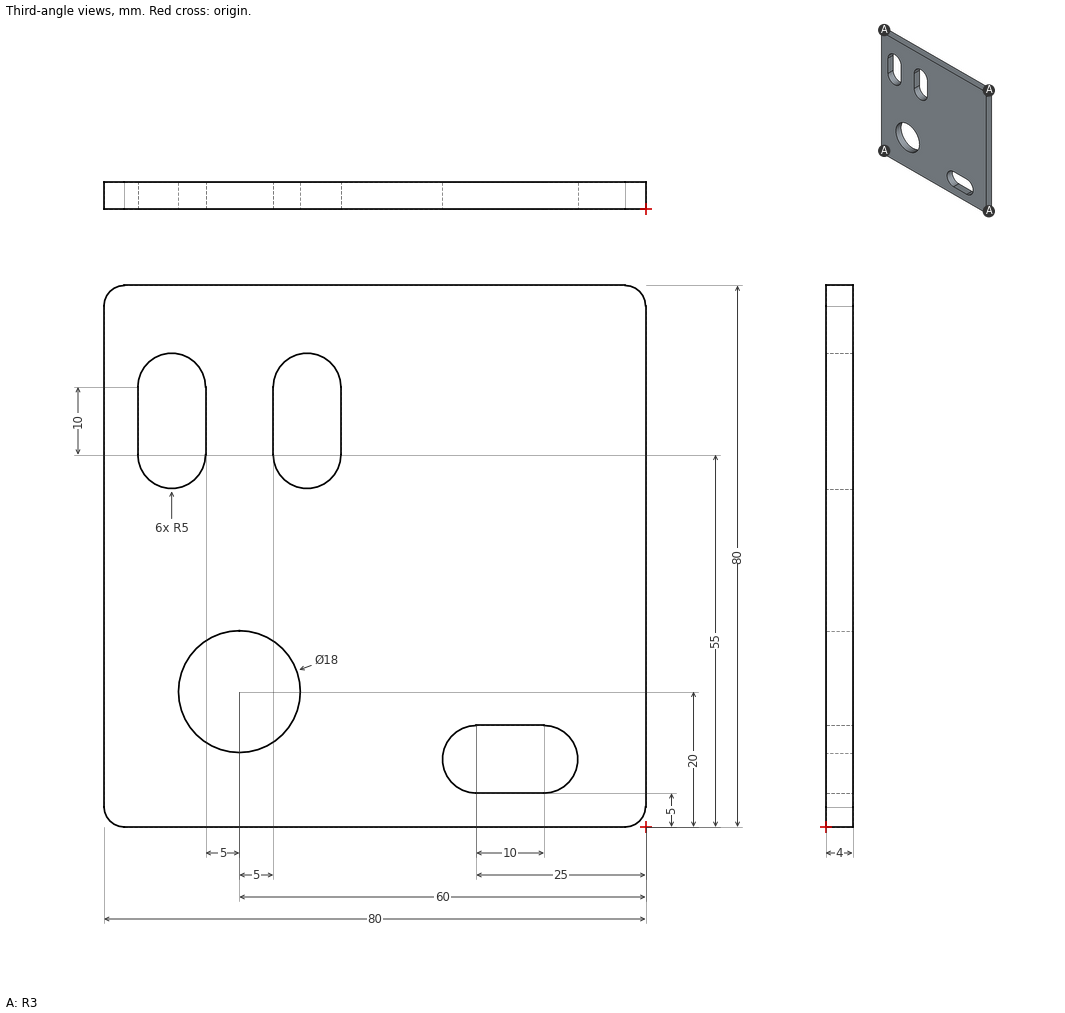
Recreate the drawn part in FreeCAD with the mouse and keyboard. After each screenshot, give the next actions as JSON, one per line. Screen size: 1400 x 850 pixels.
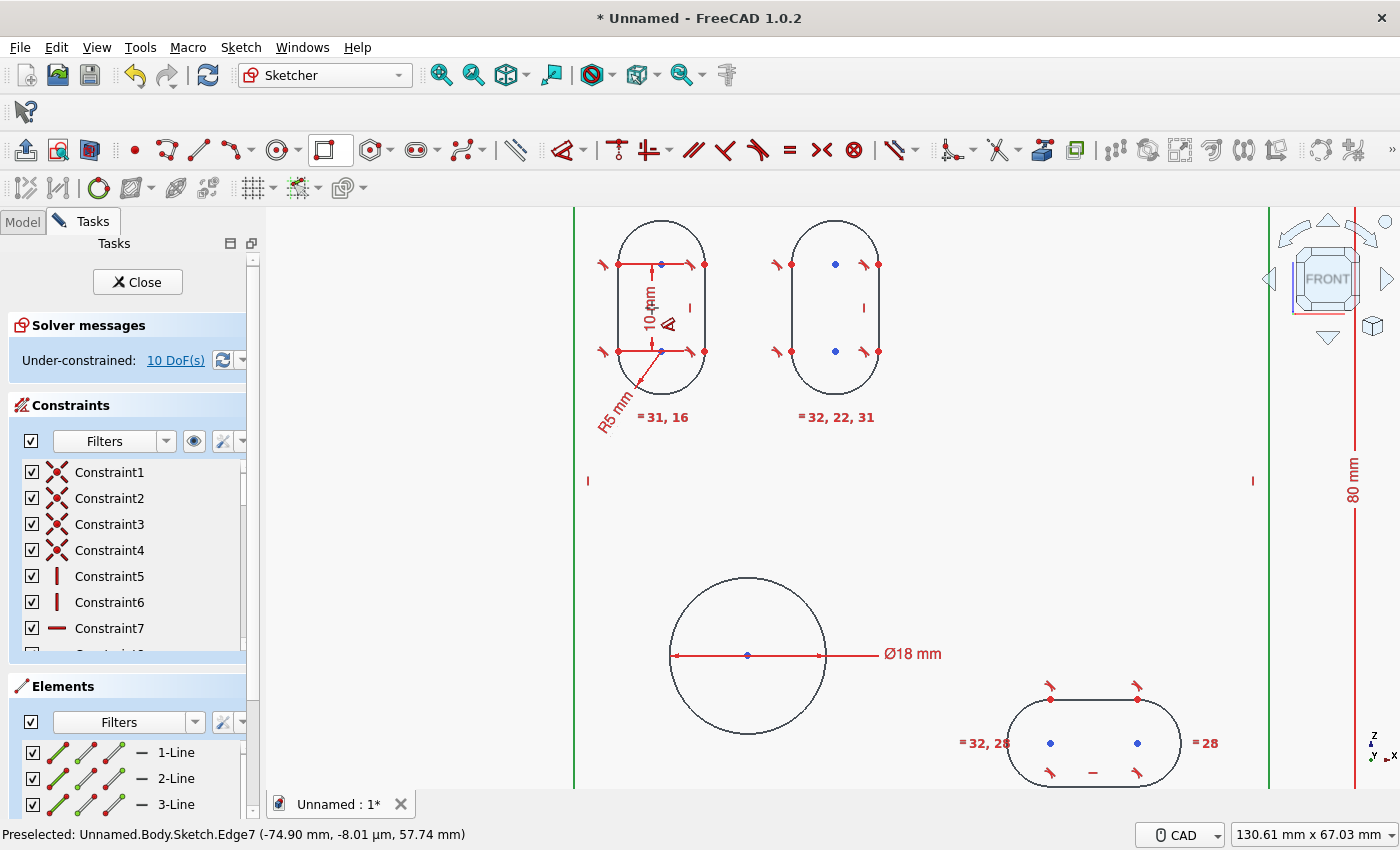
{"action": "left_click", "coordinate": [792, 325]}
{"action": "left_click", "coordinate": [758, 308]}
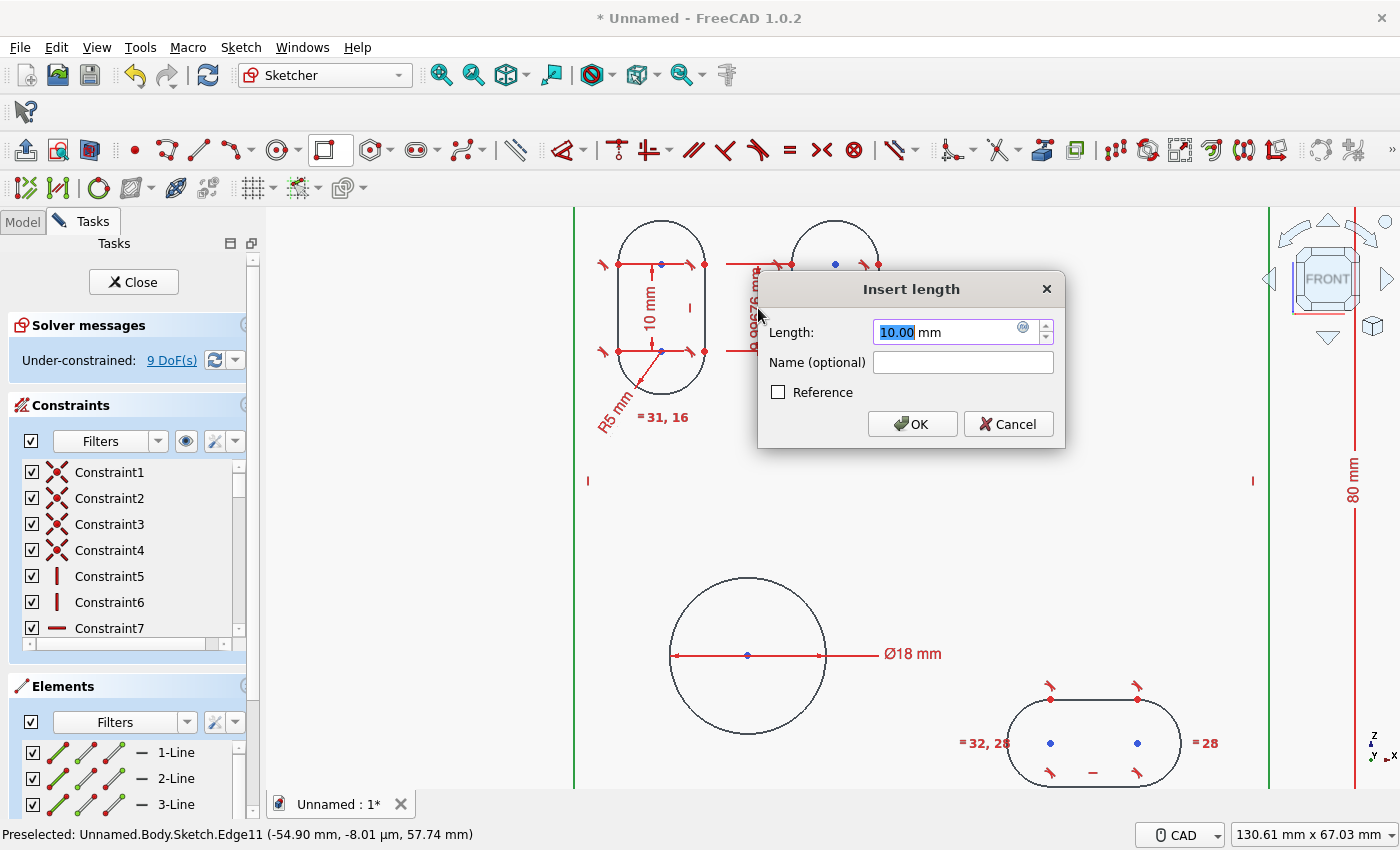
{"action": "type", "text": "10"}
{"action": "key", "text": "Return"}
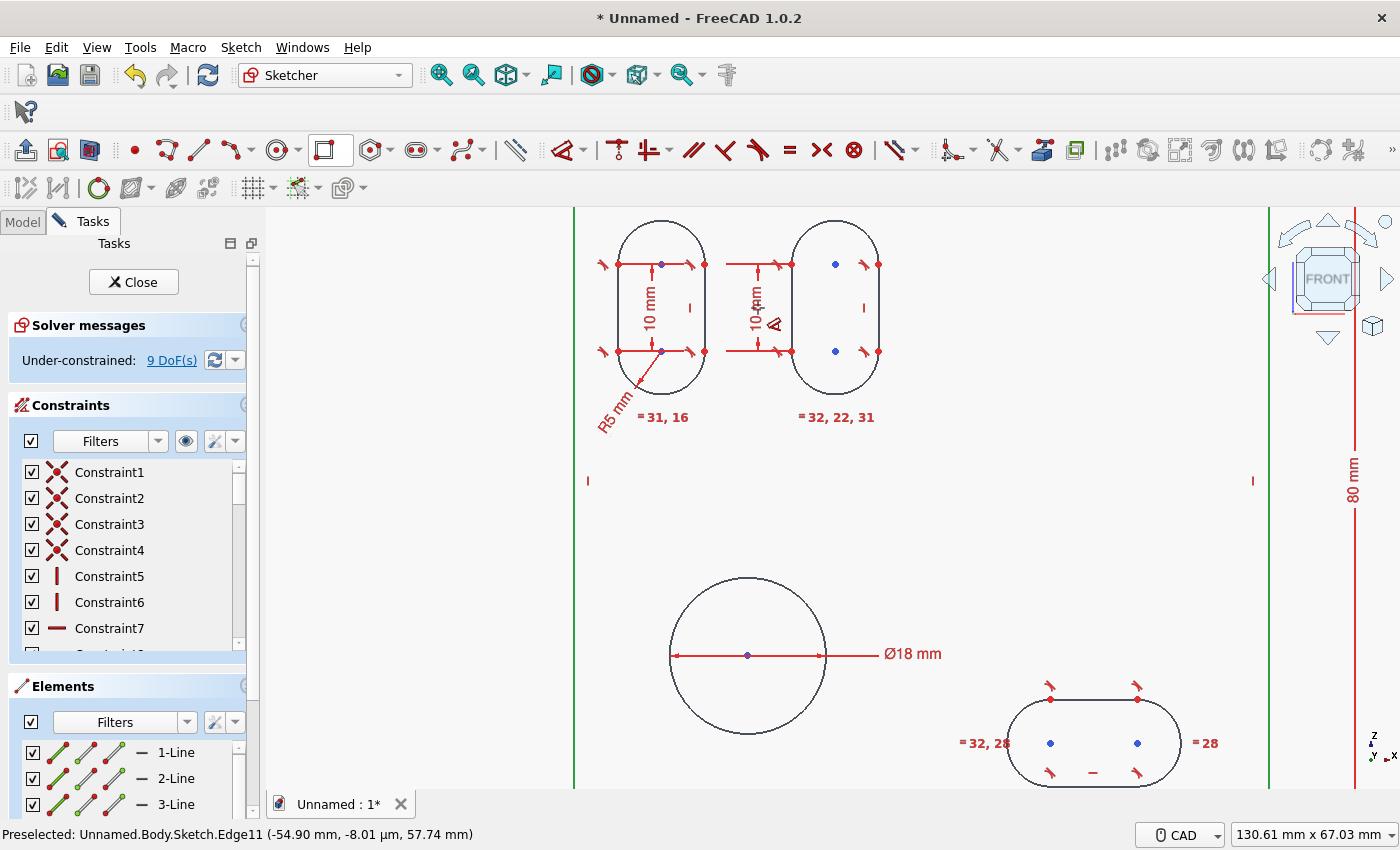
{"action": "left_click", "coordinate": [1077, 700]}
{"action": "left_click", "coordinate": [1094, 734]}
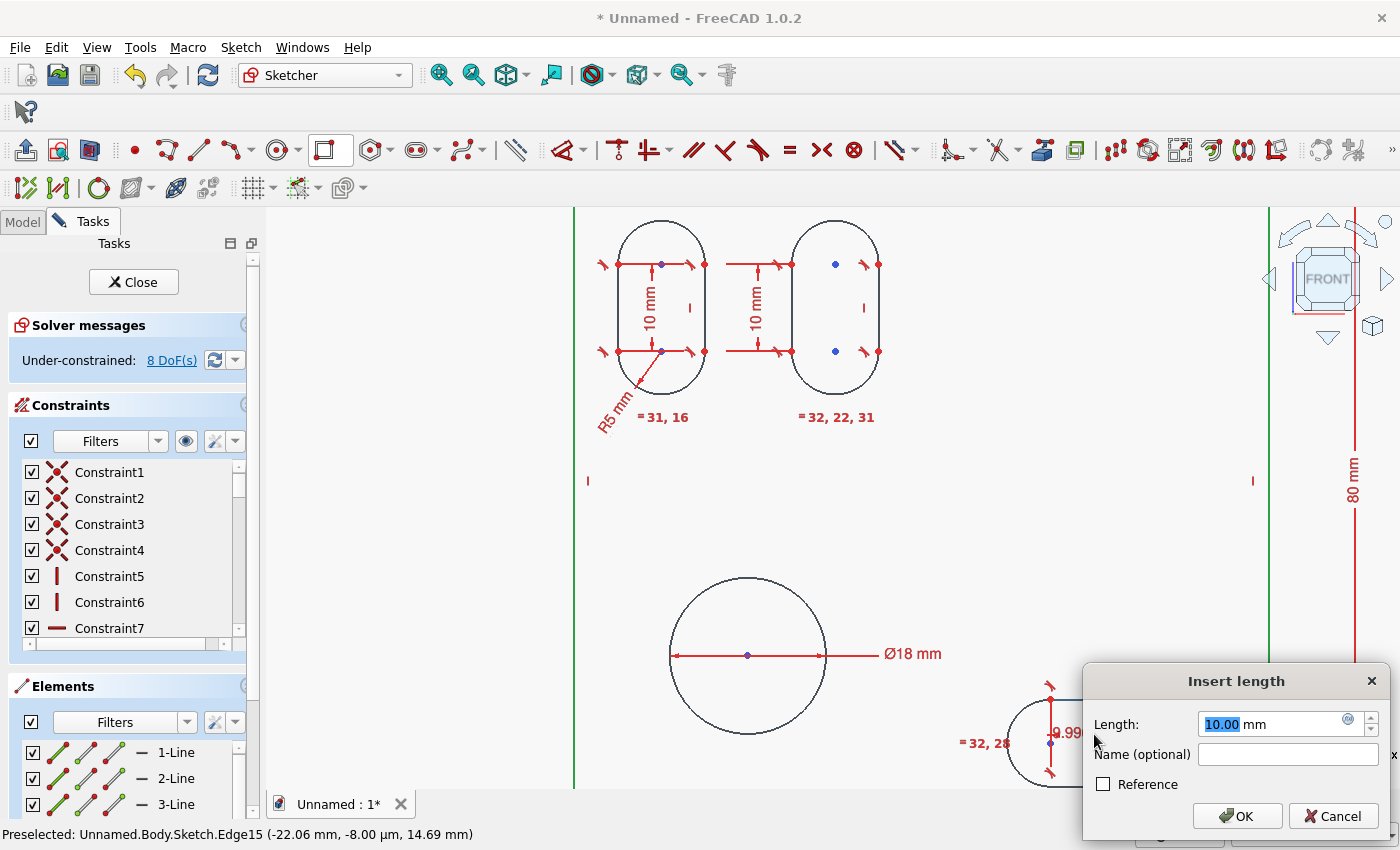
{"action": "type", "text": "10"}
{"action": "key", "text": "Return"}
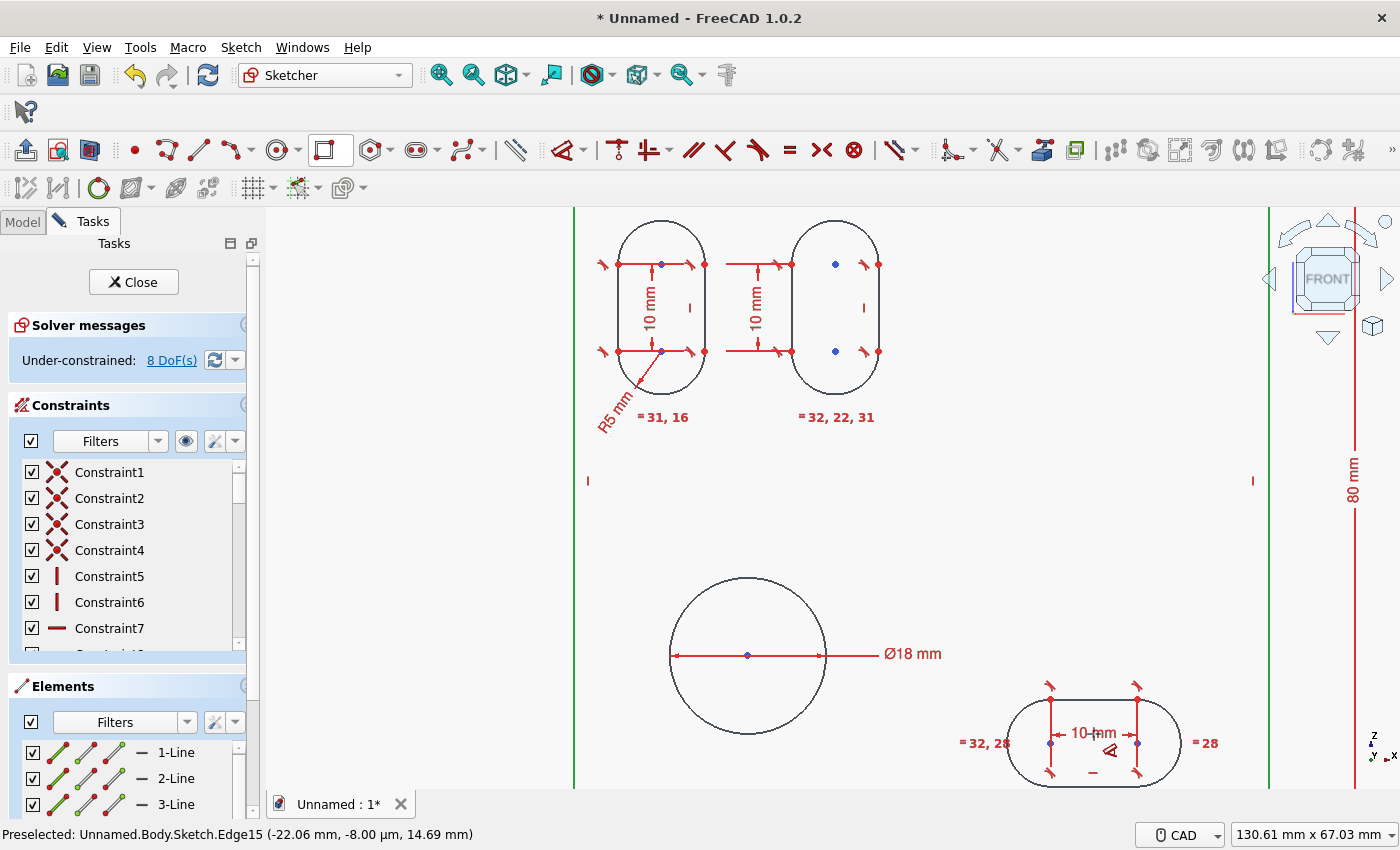
{"action": "scroll", "coordinate": [574, 520], "scroll_direction": "down", "scroll_amount": 3}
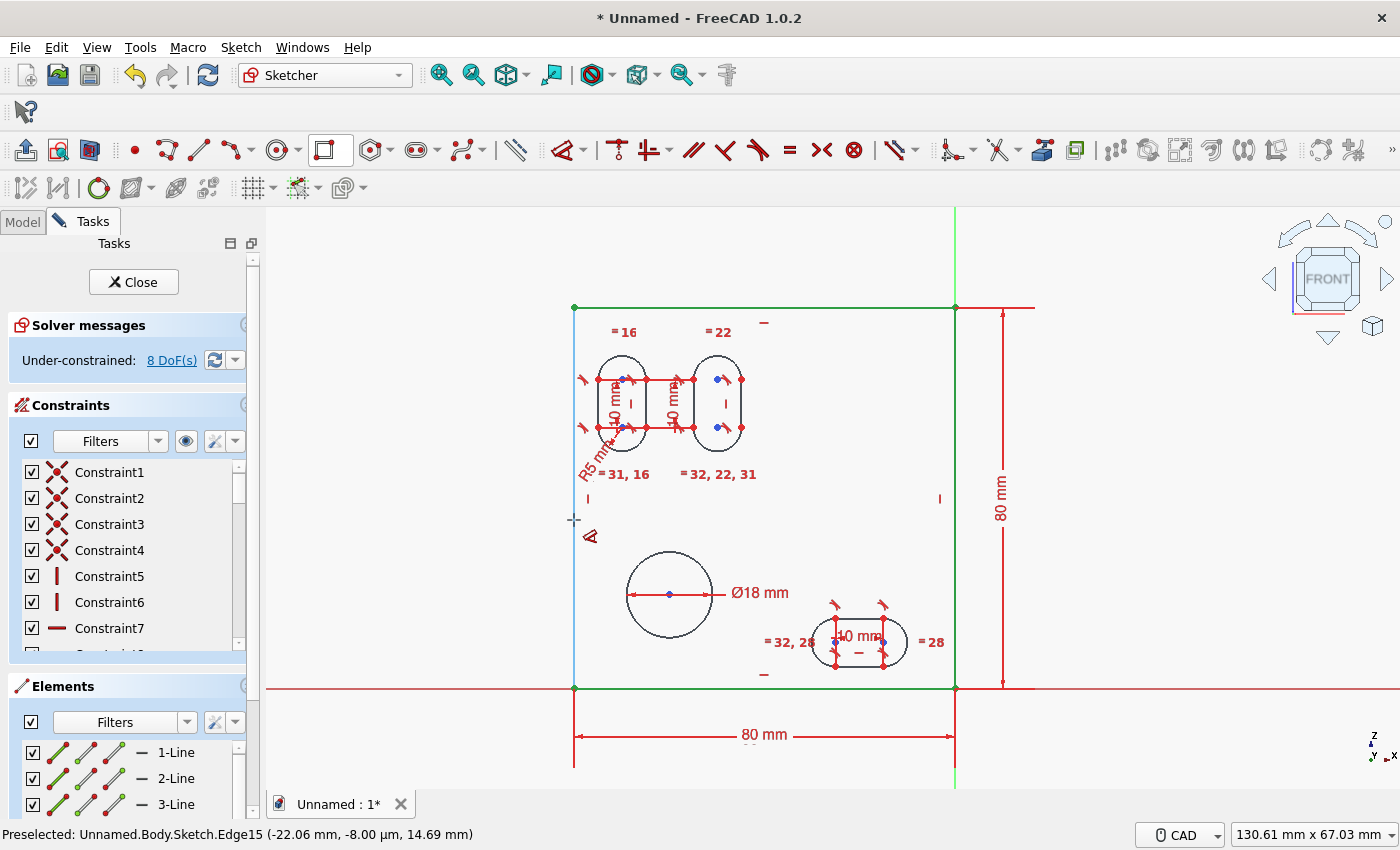
{"action": "scroll", "coordinate": [836, 667], "scroll_direction": "up", "scroll_amount": 3}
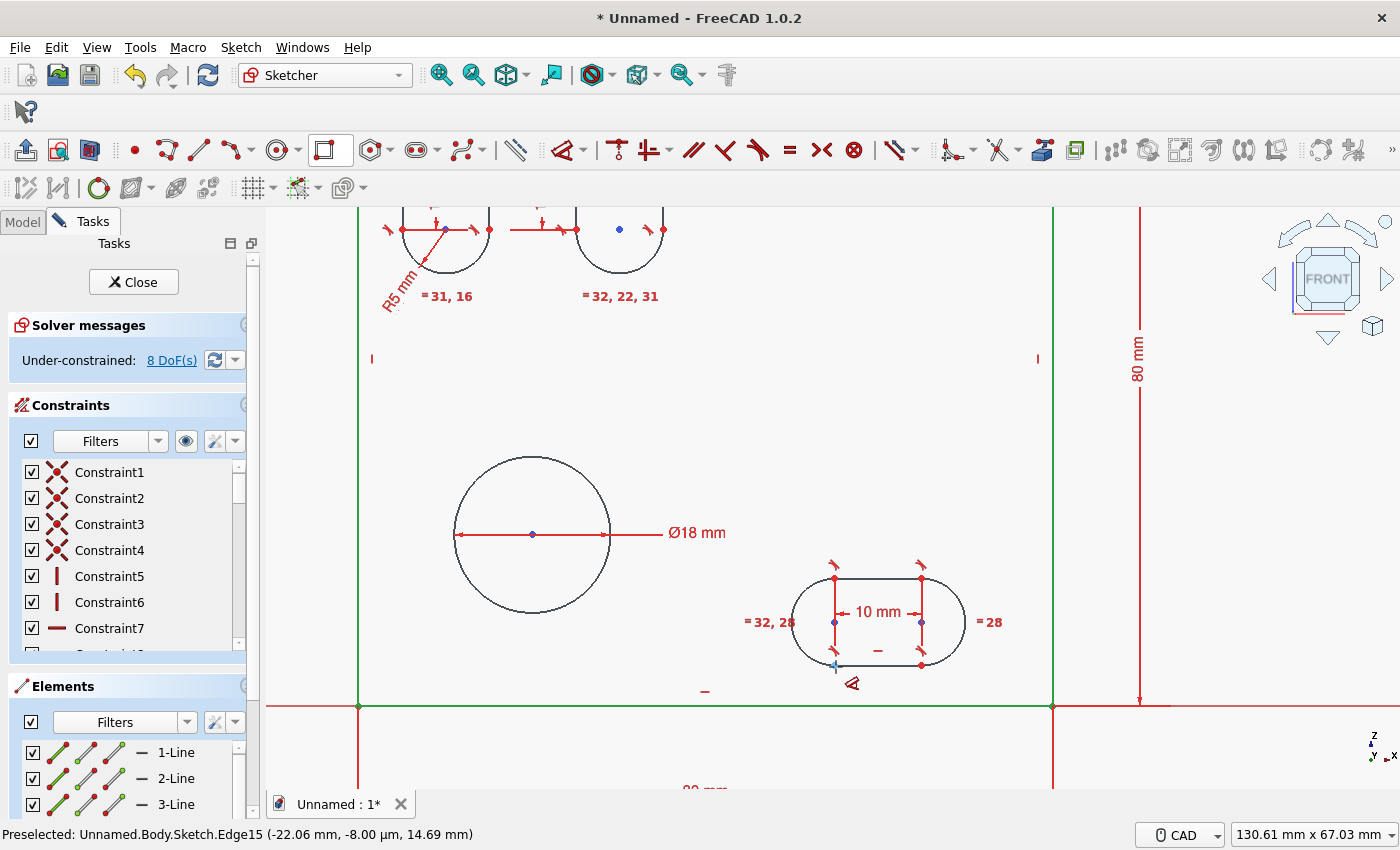
{"action": "left_click", "coordinate": [835, 666]}
{"action": "left_click", "coordinate": [1087, 686]}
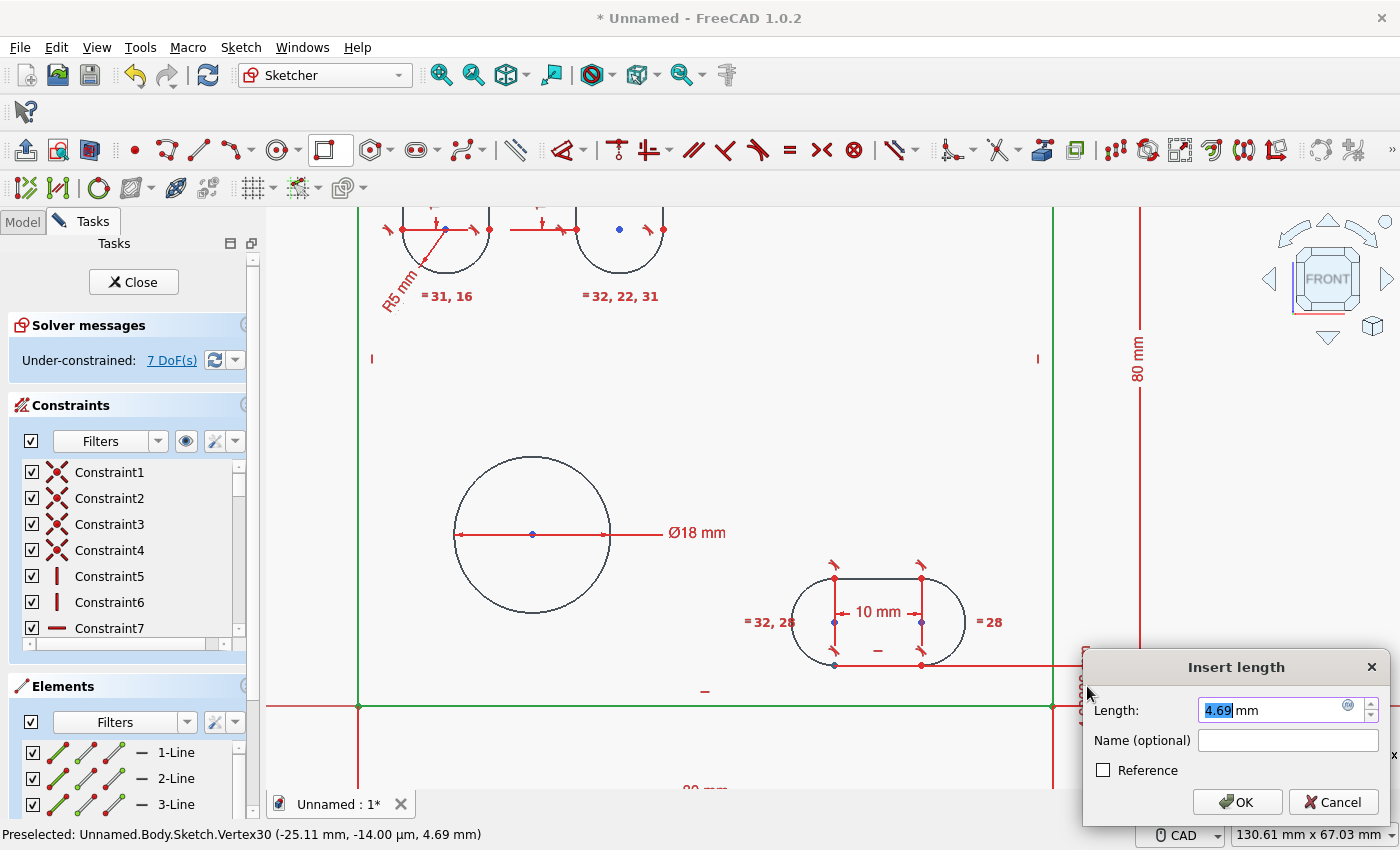
{"action": "type", "text": "5"}
{"action": "key", "text": "Return"}